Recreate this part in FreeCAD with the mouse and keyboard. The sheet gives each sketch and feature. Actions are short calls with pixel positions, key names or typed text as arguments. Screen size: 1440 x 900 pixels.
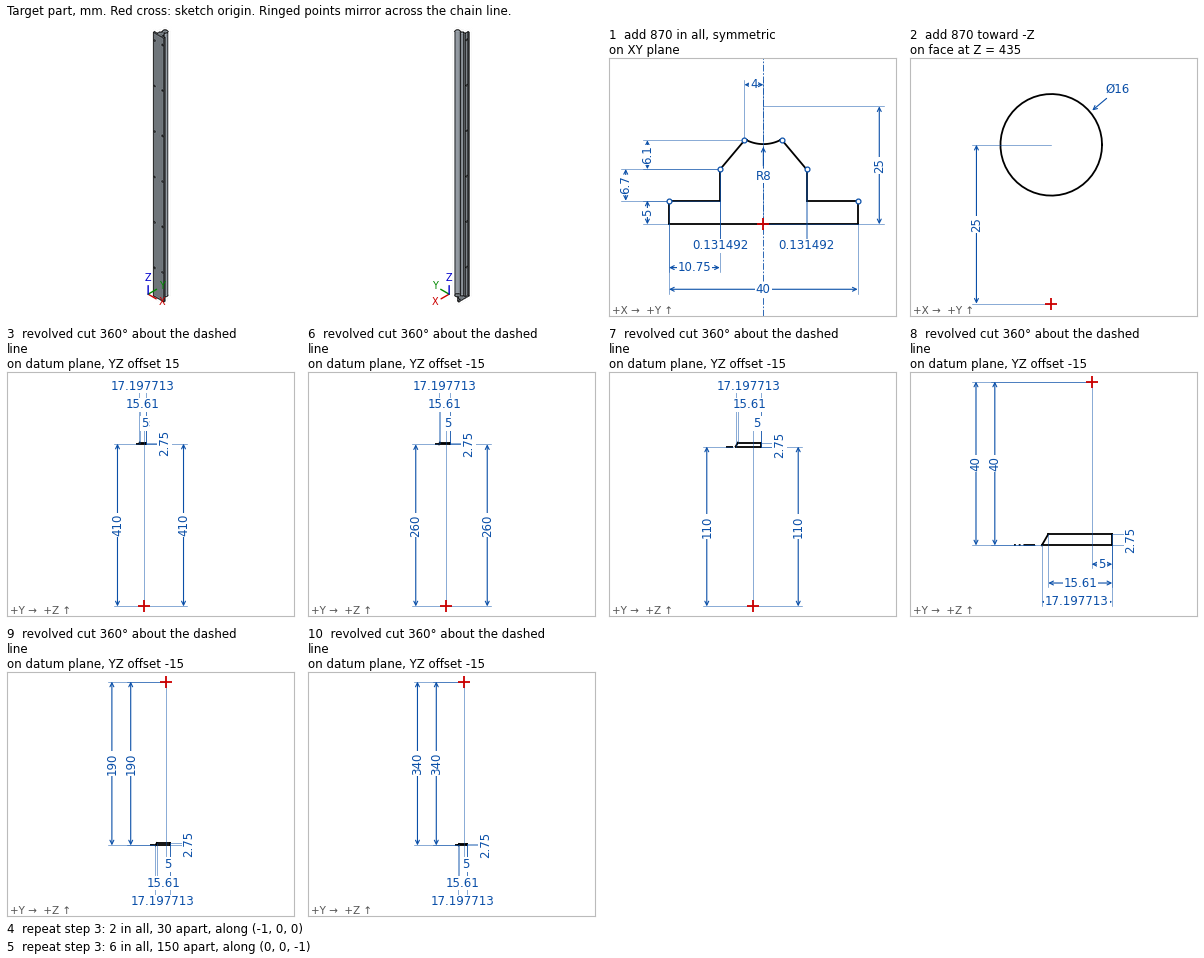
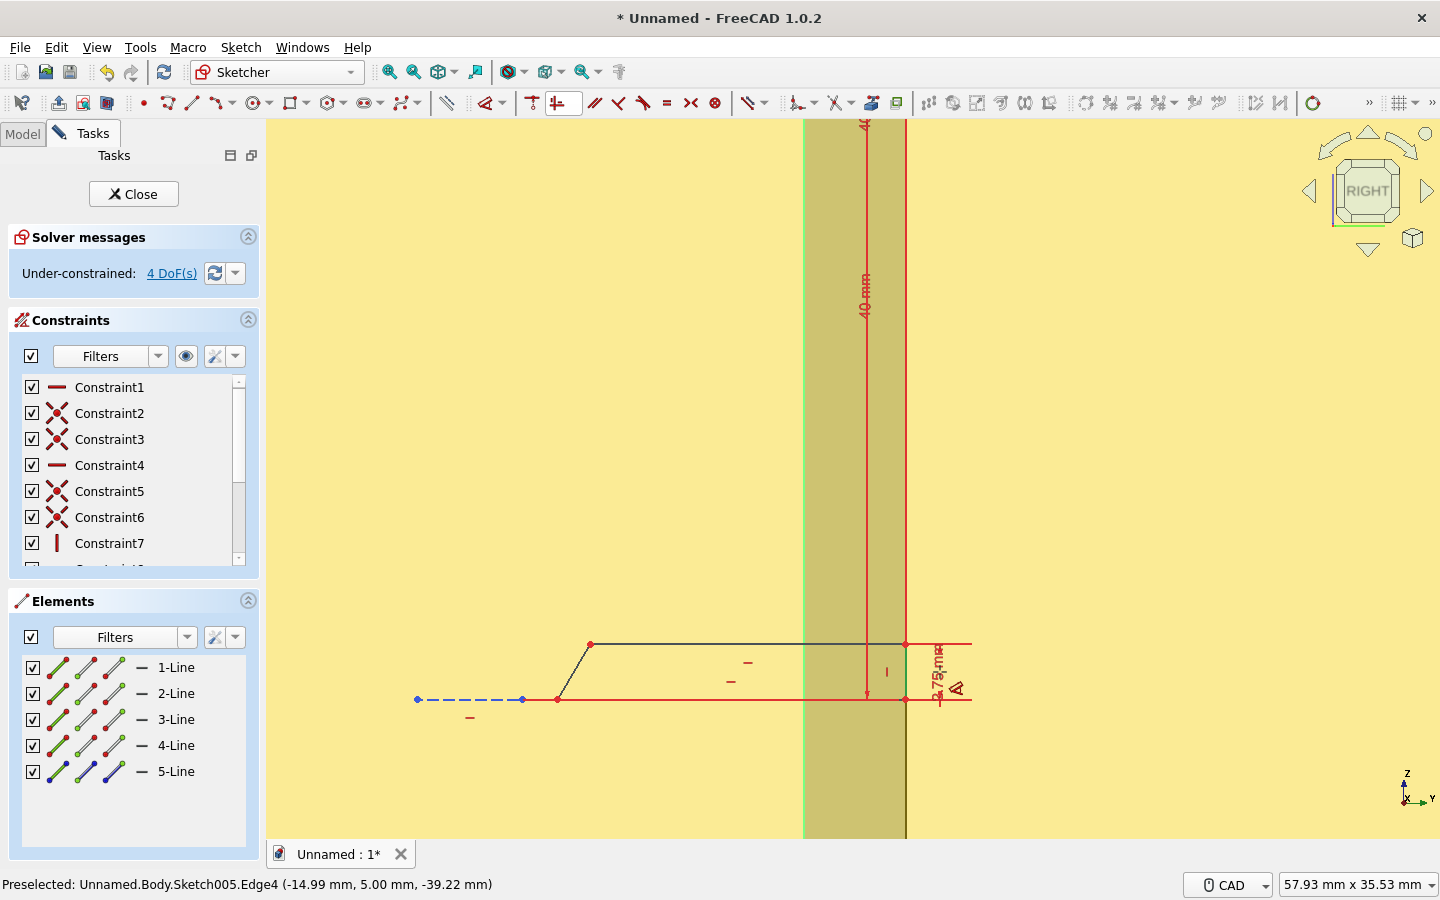
click(685, 644)
click(748, 678)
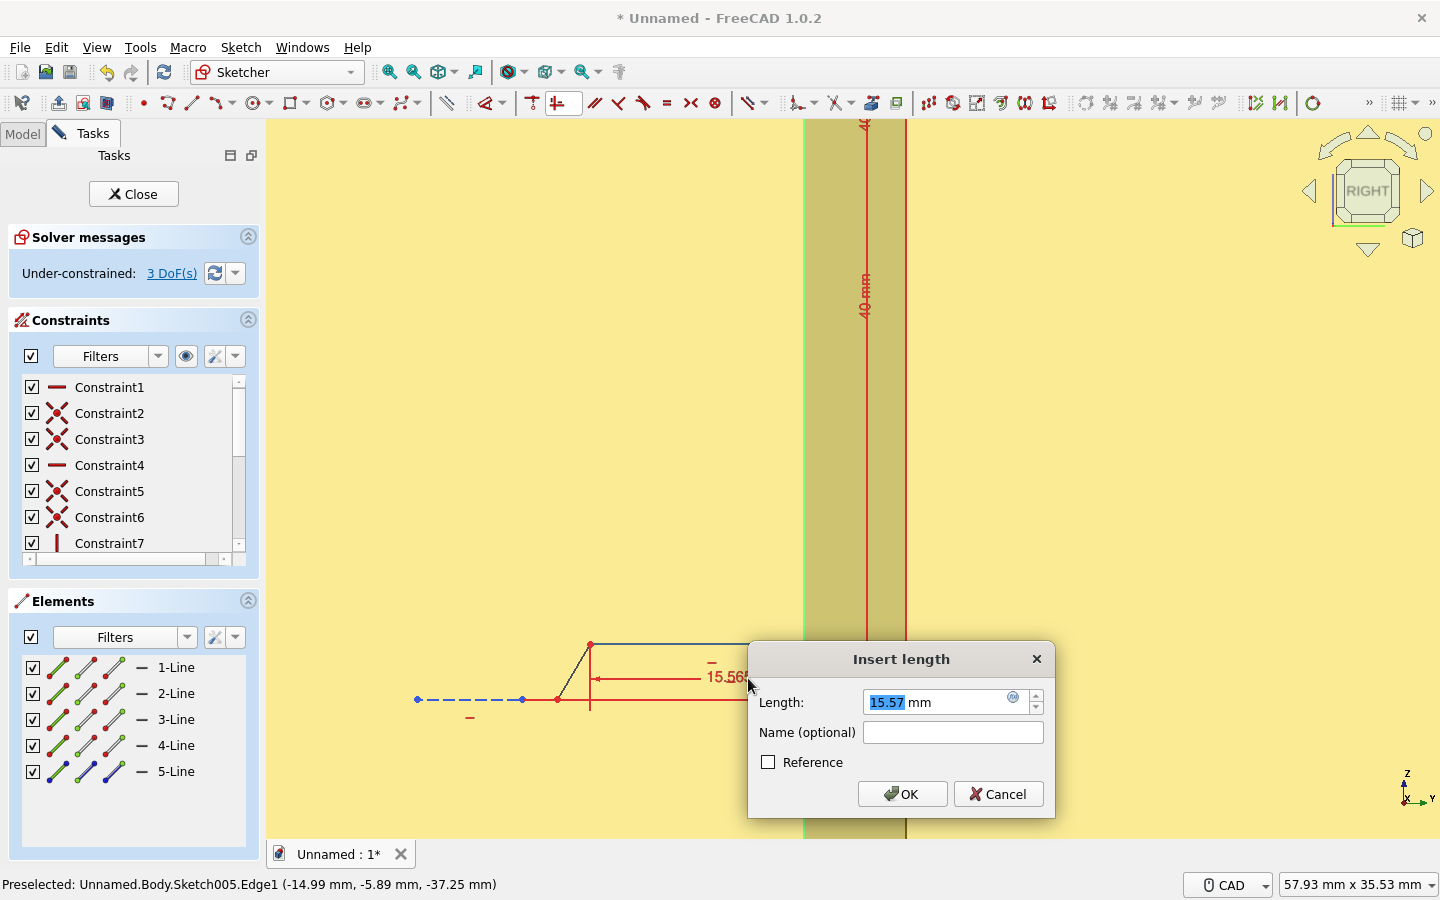
text(15.61)
key(Return)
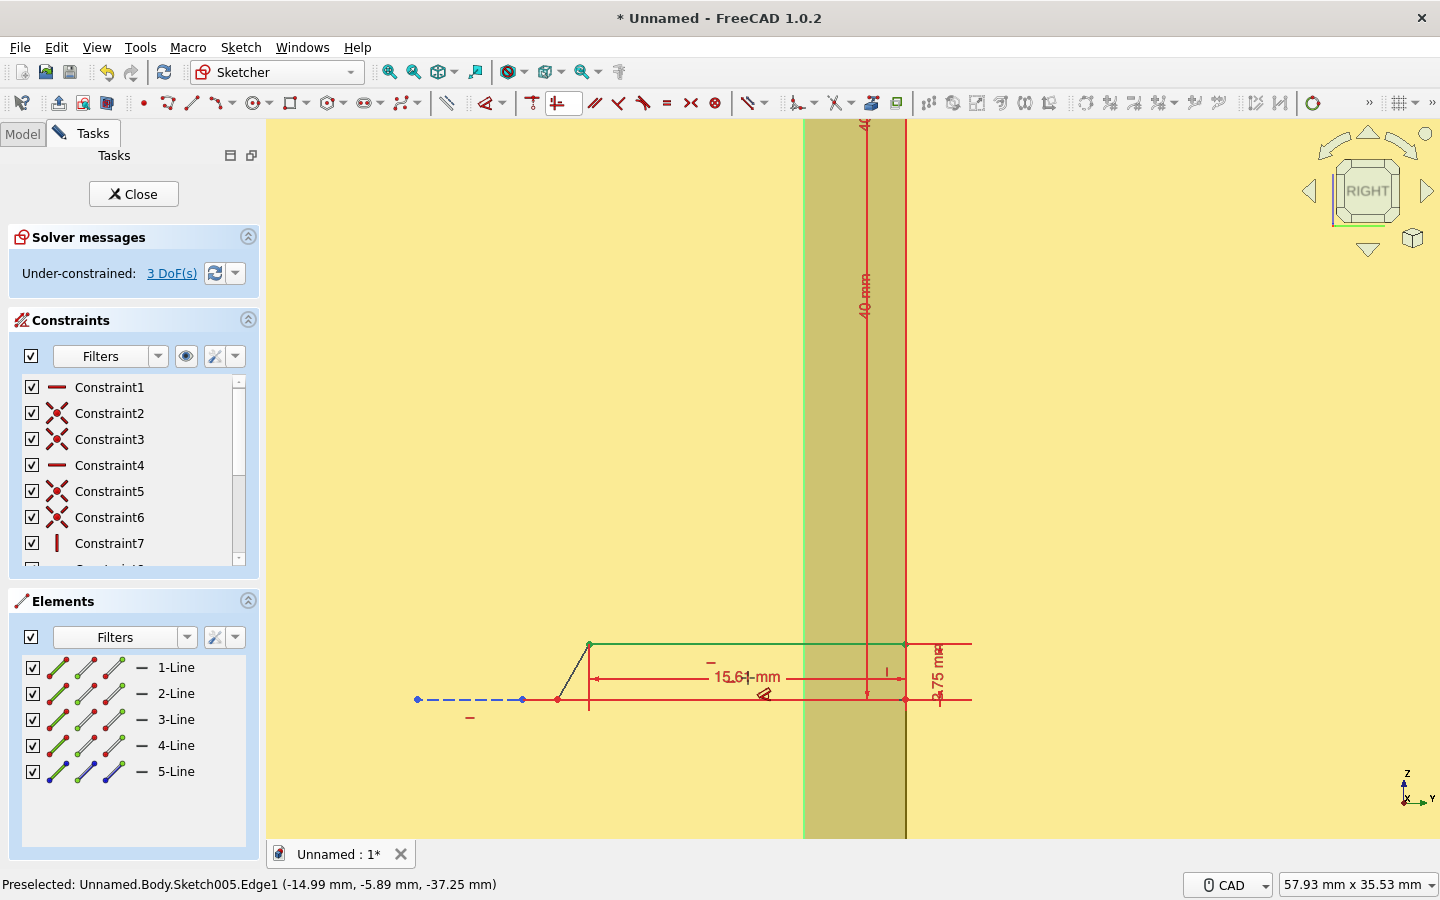
click(662, 700)
click(732, 734)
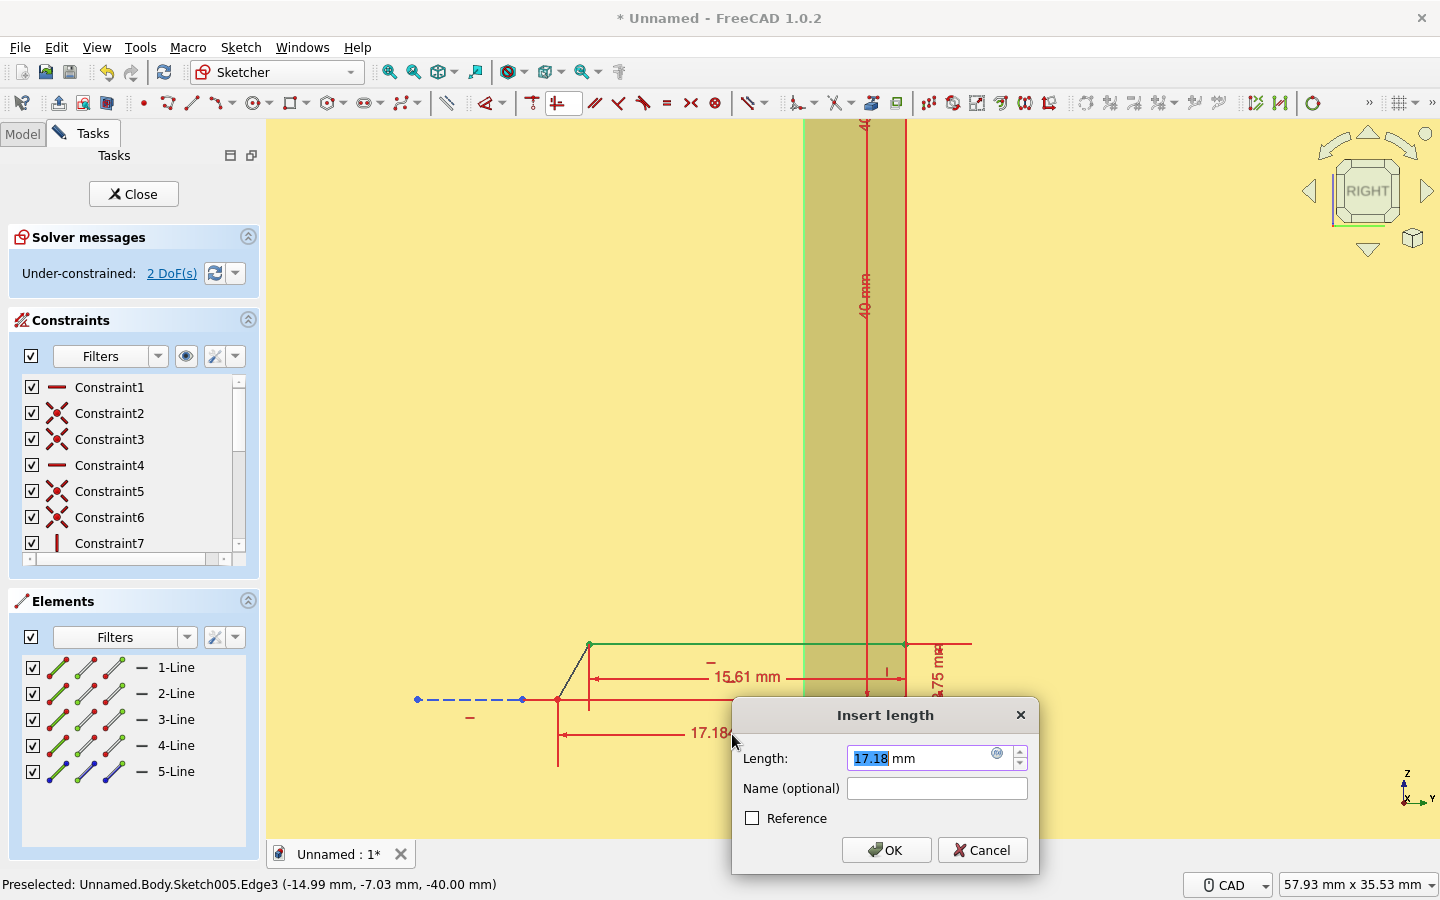
text(17.197713)
key(Return)
key(Escape)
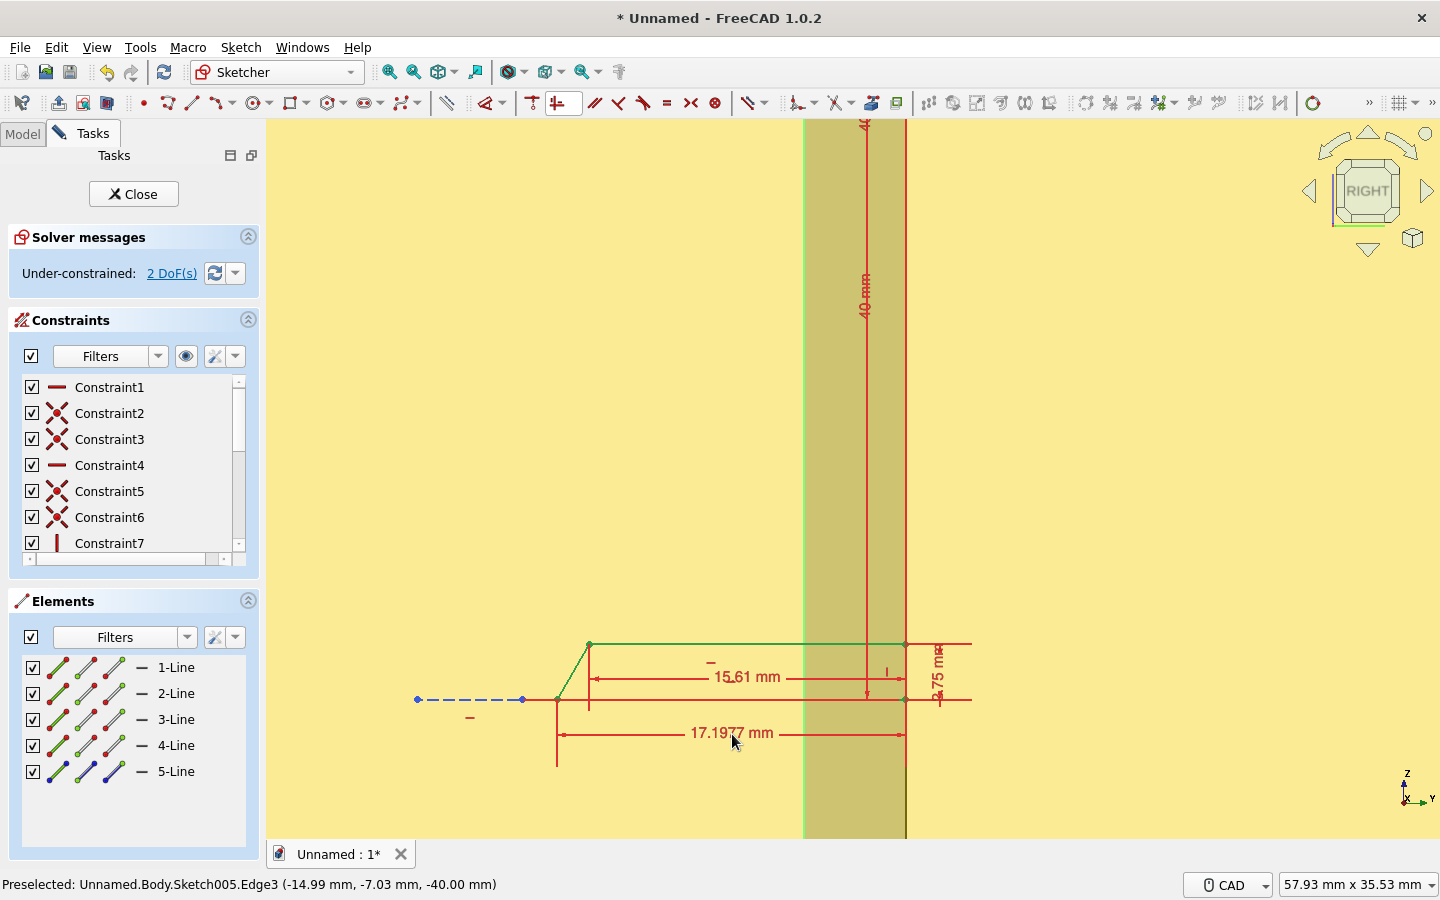
click(134, 194)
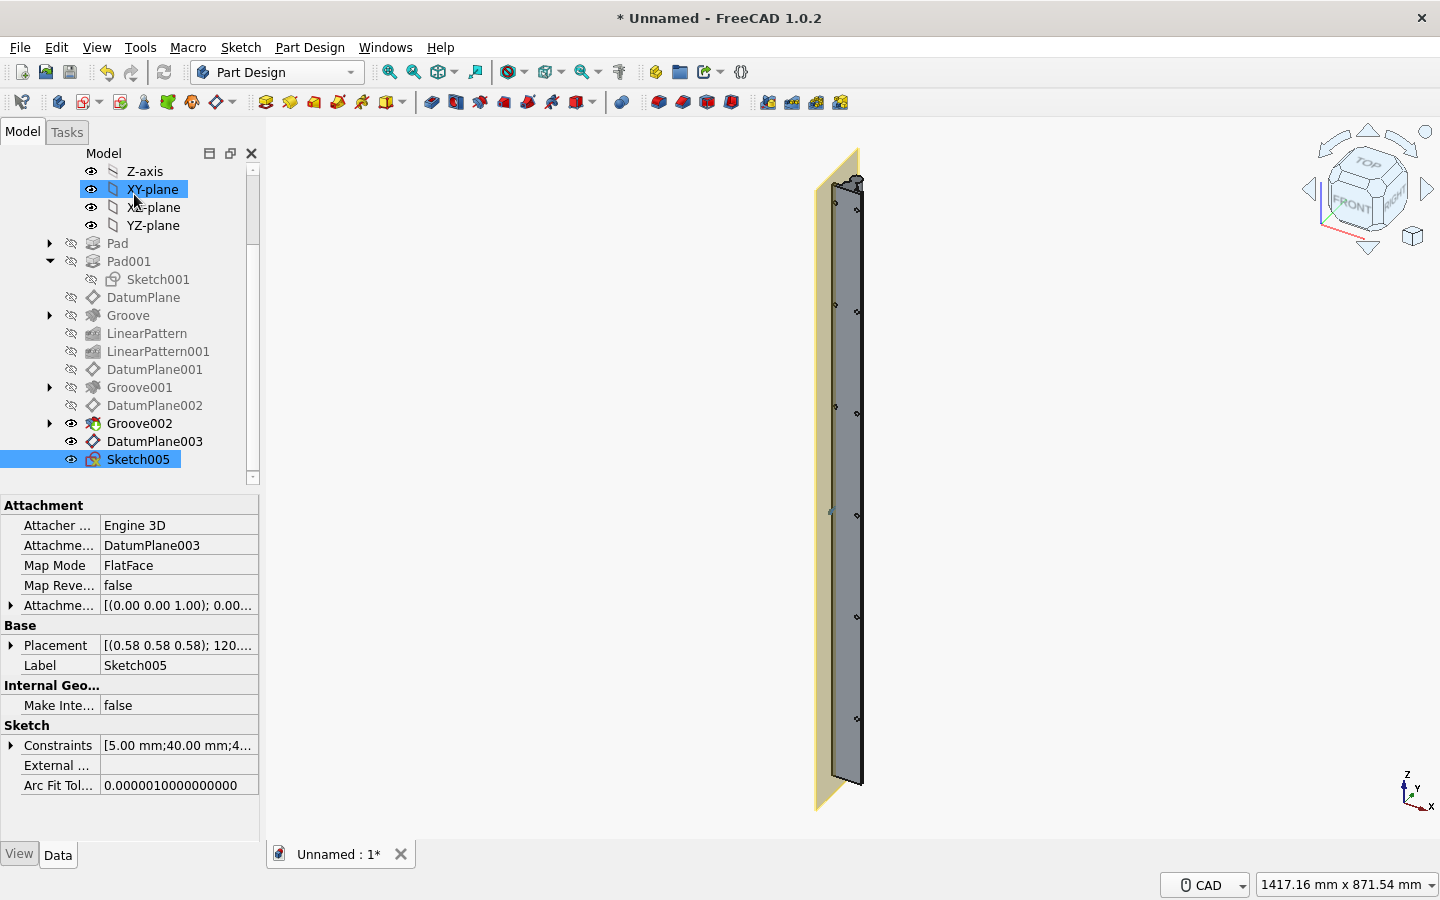
click(480, 102)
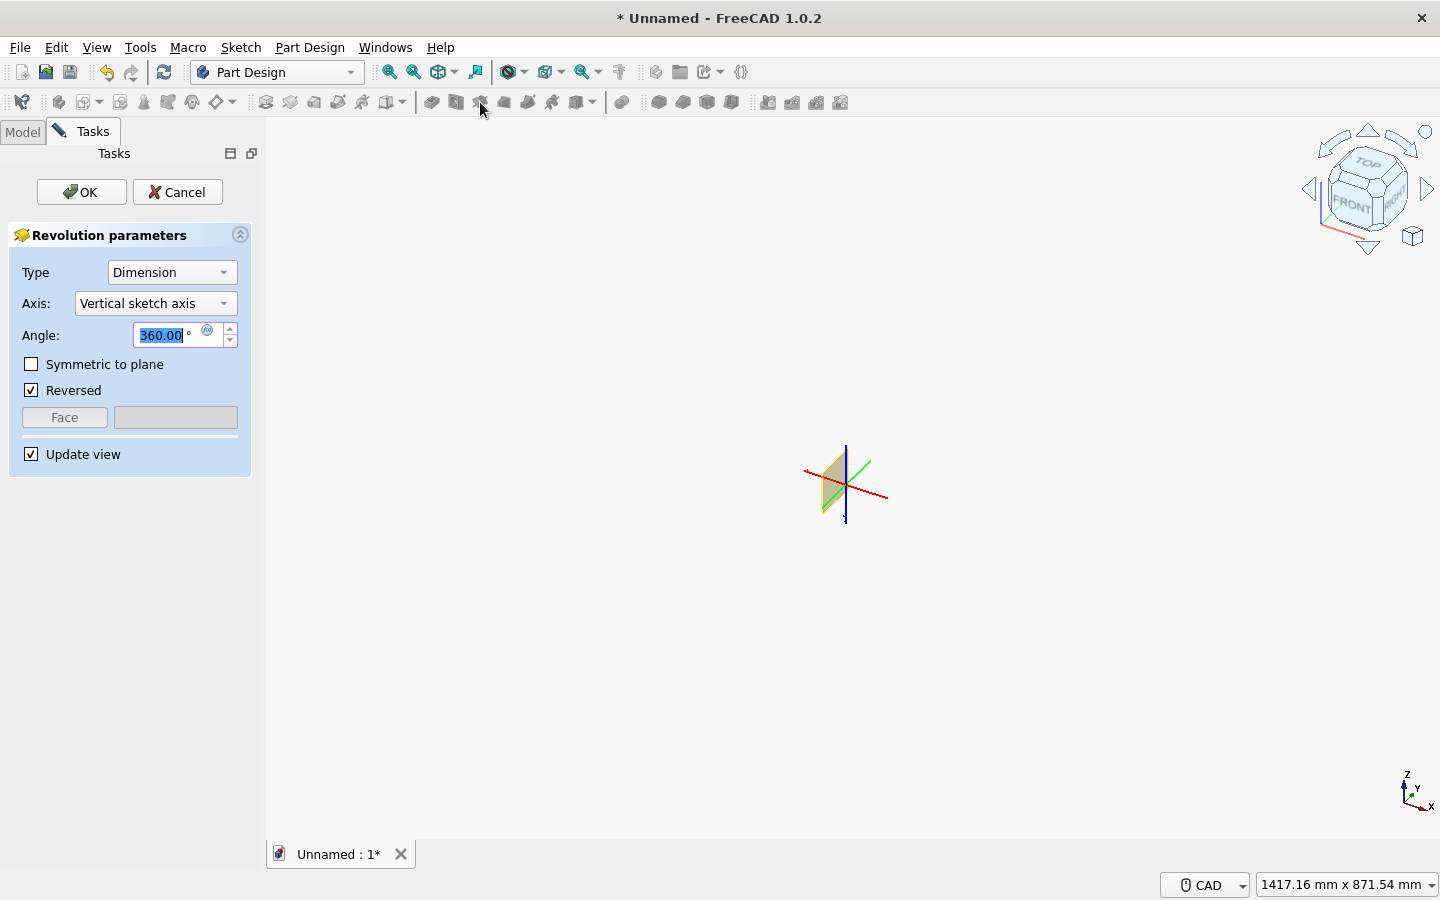
click(156, 304)